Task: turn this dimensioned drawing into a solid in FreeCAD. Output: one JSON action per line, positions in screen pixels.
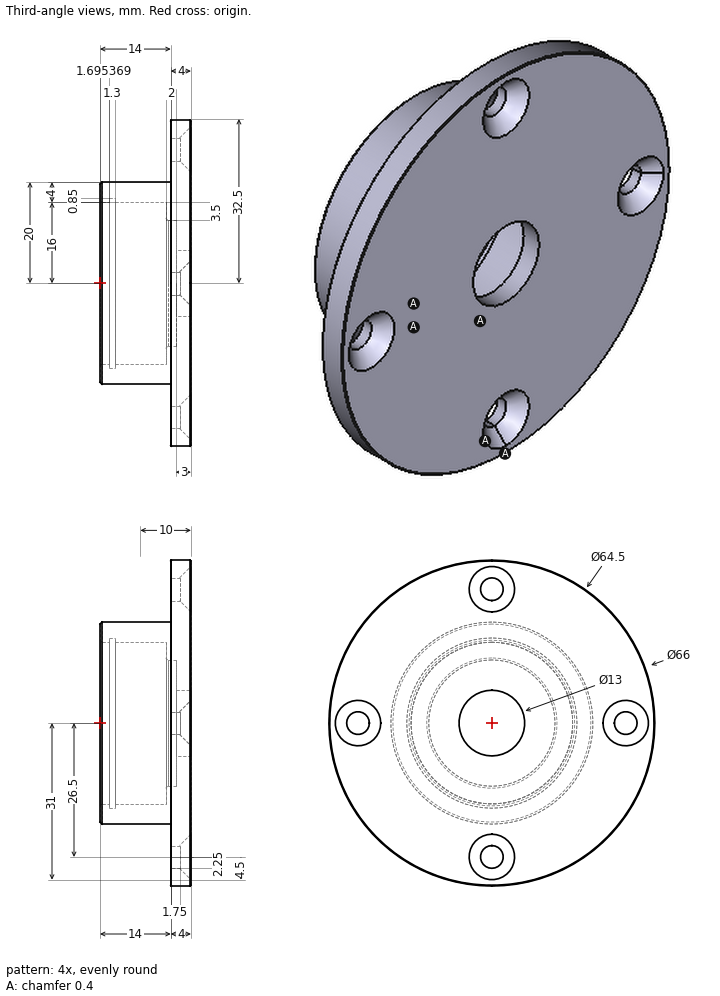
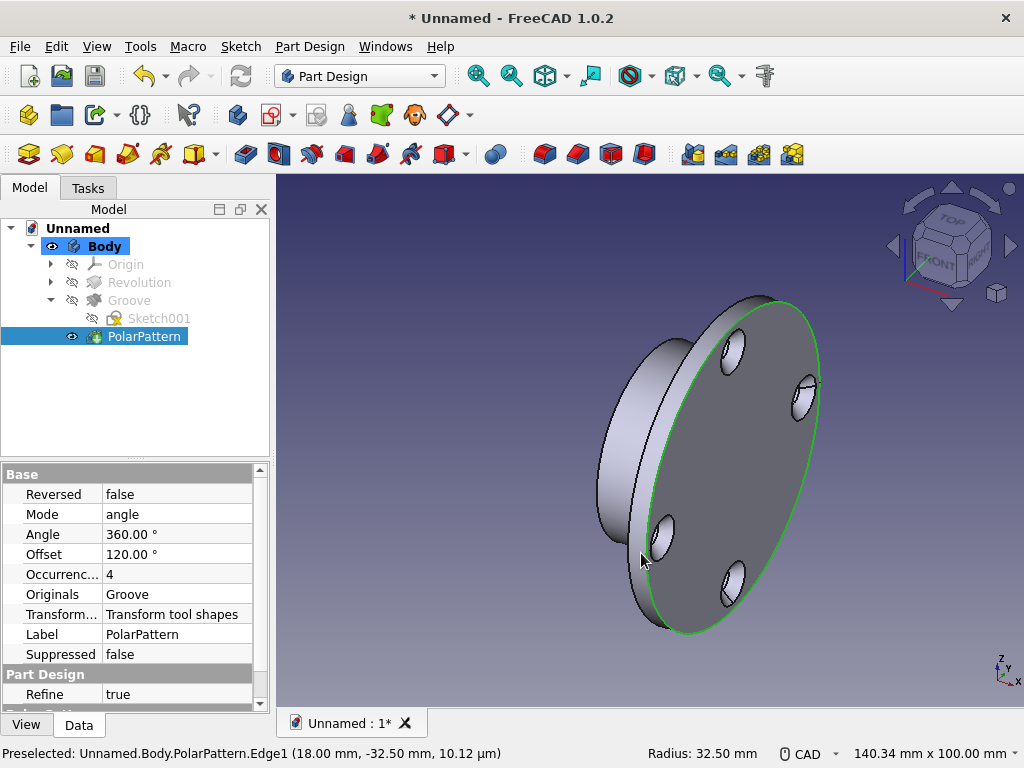
{"action": "key", "text": "0"}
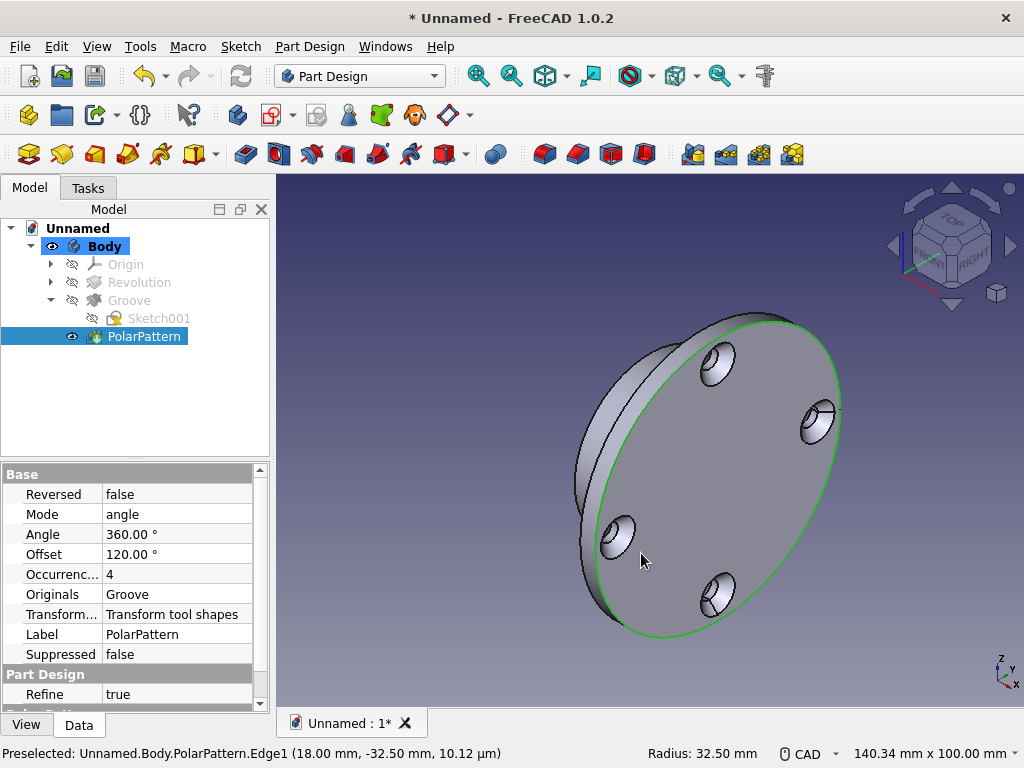
{"action": "key", "text": "2"}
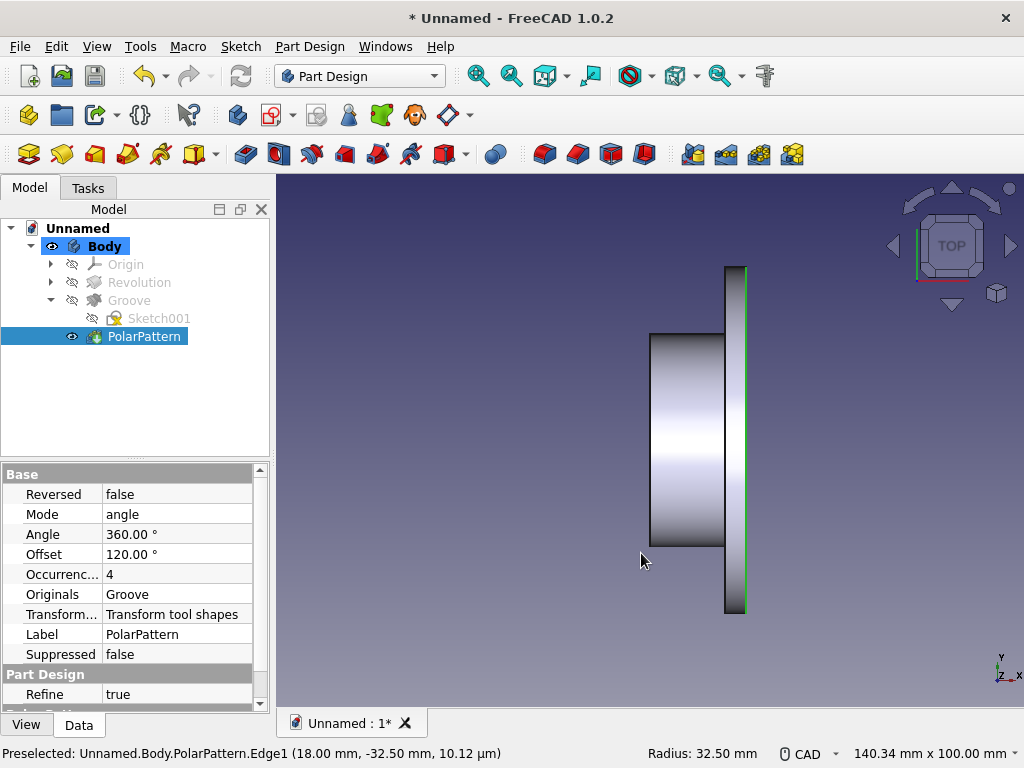
{"action": "left_click", "coordinate": [725, 580], "text": "ctrl"}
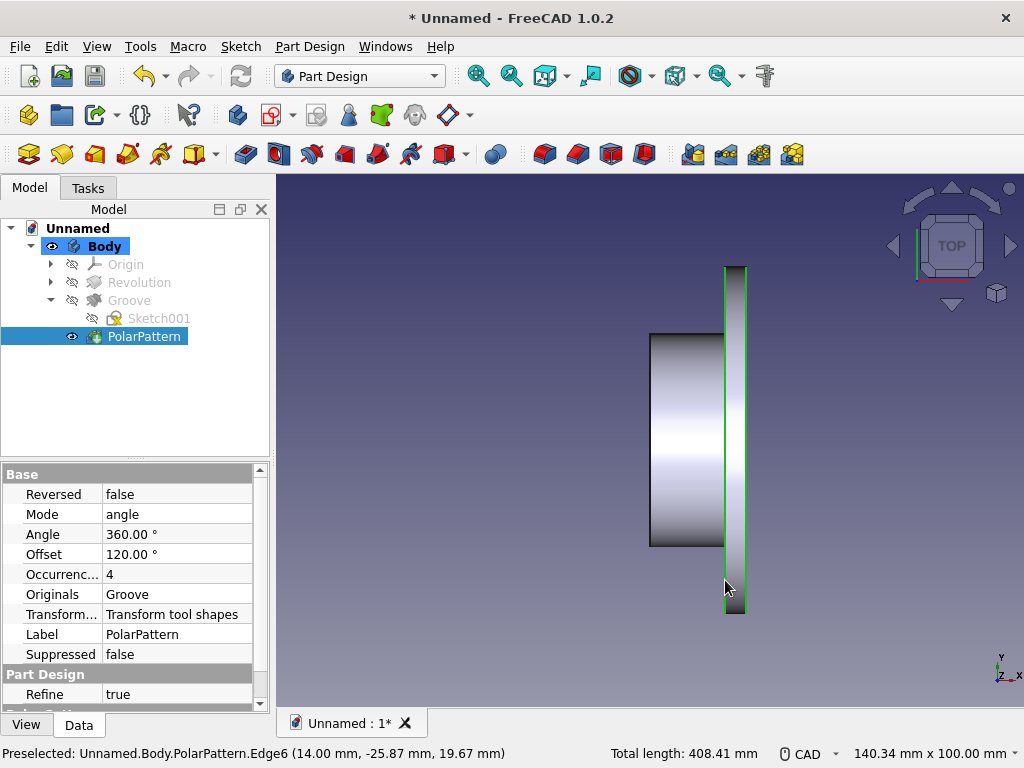
{"action": "left_click", "coordinate": [650, 526], "text": "ctrl"}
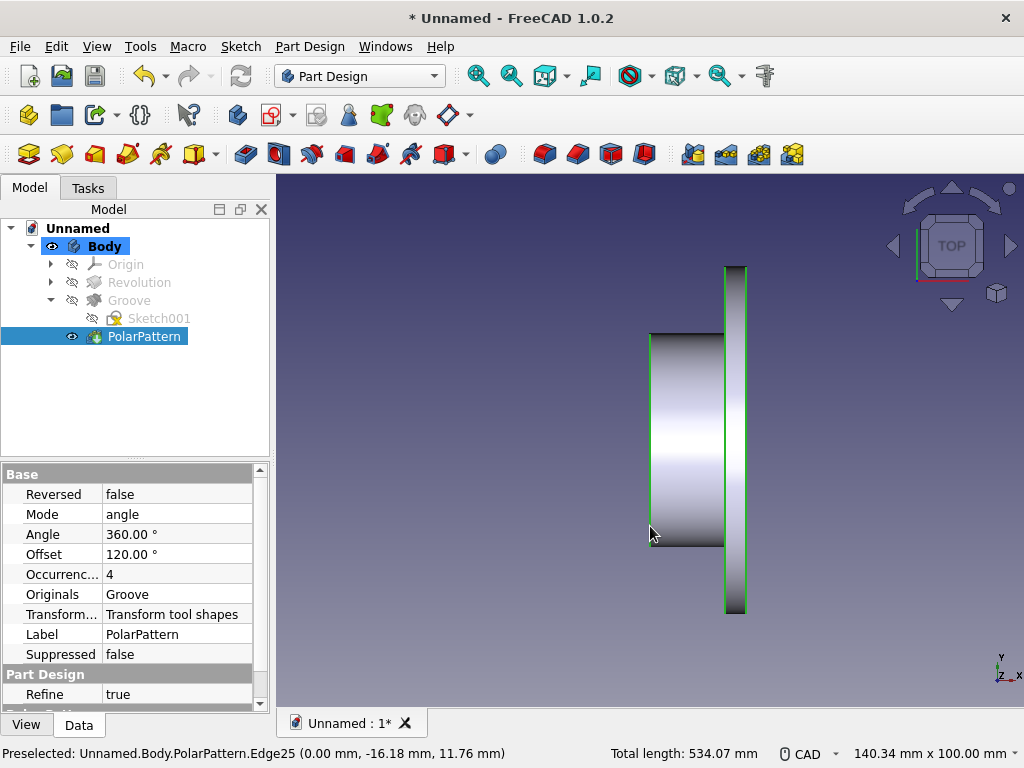
{"action": "key", "text": "1"}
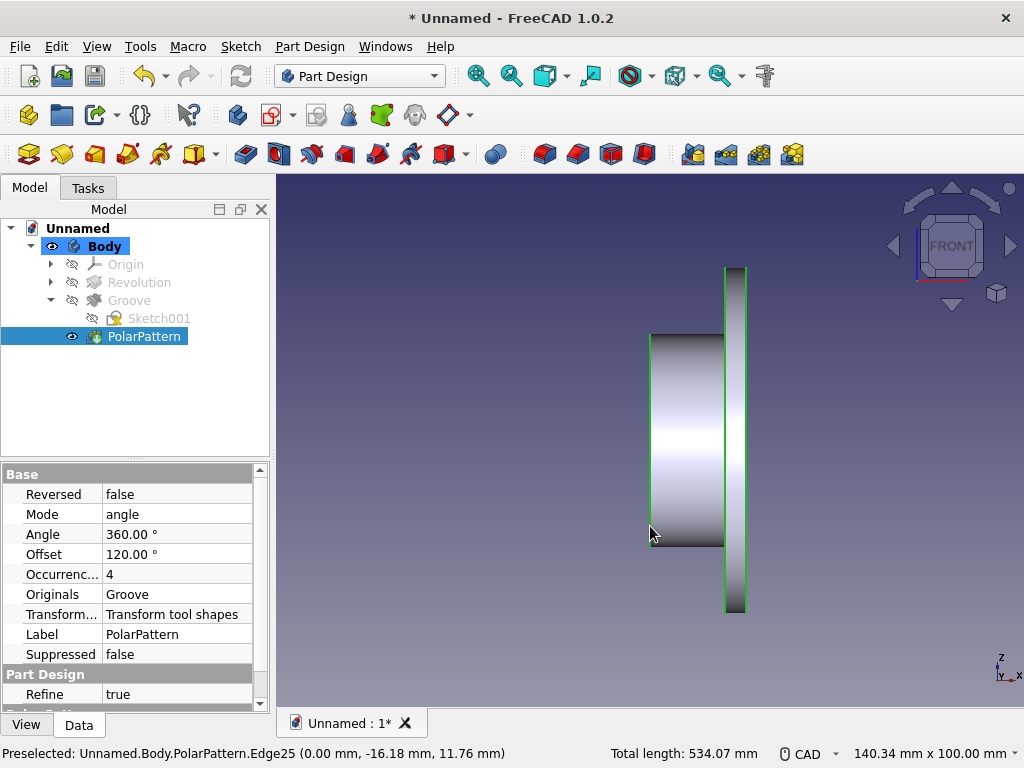
{"action": "key", "text": "3"}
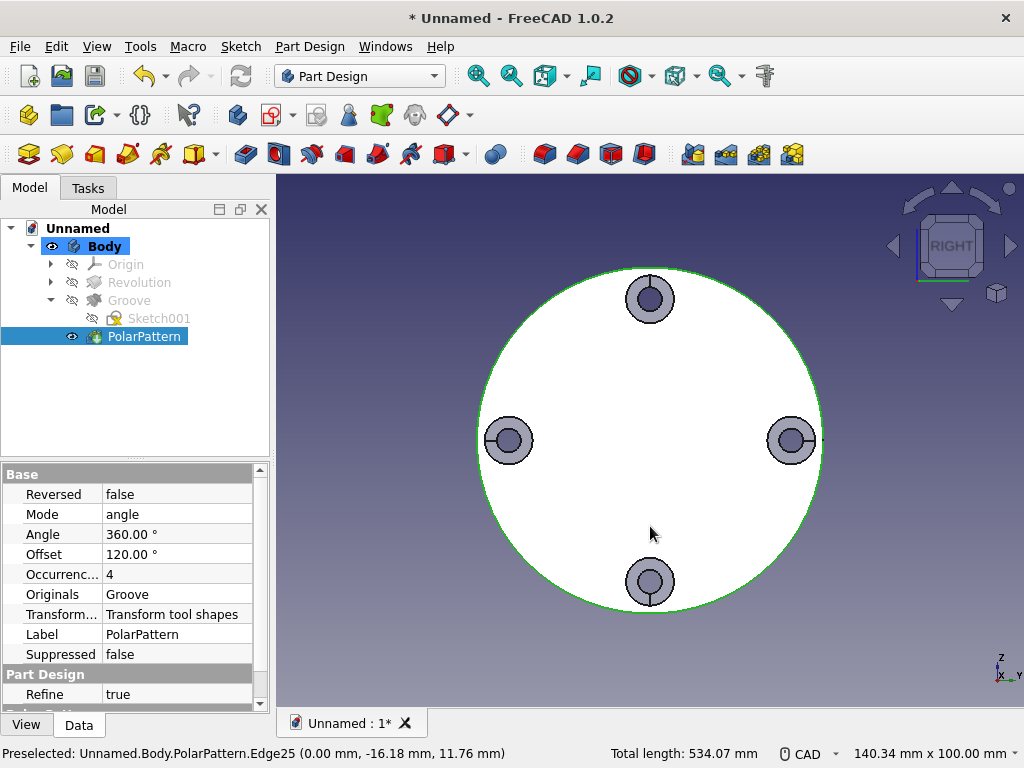
{"action": "key", "text": "5"}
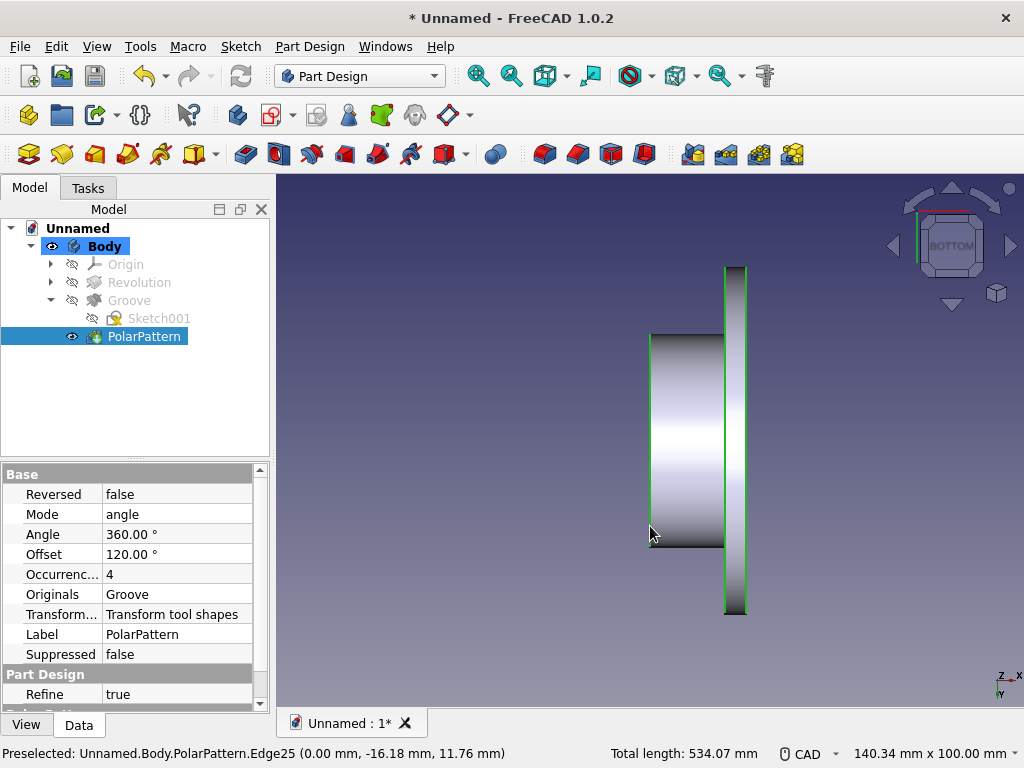
{"action": "key", "text": "4"}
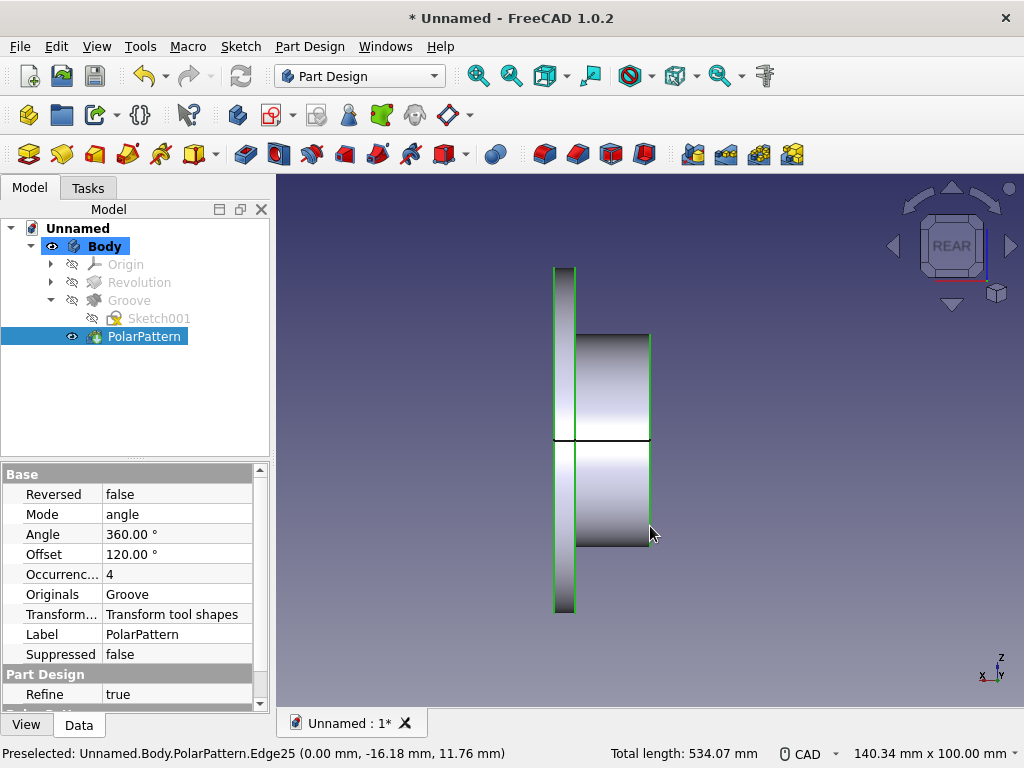
{"action": "key", "text": "6"}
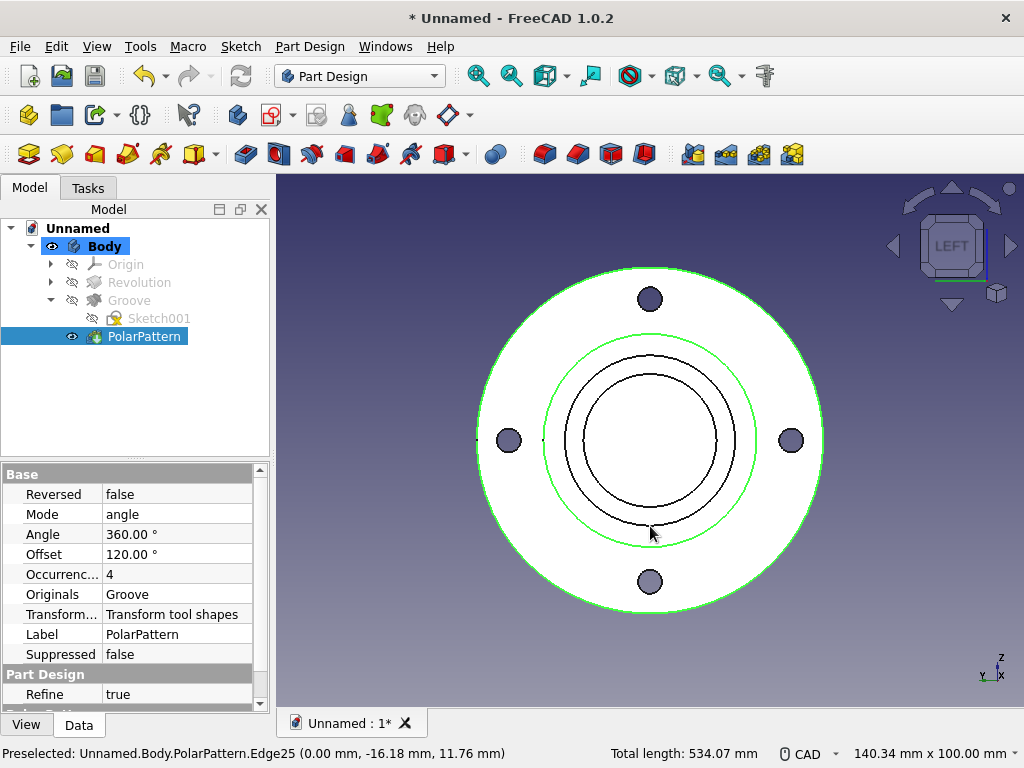
{"action": "left_click", "coordinate": [717, 439], "text": "ctrl"}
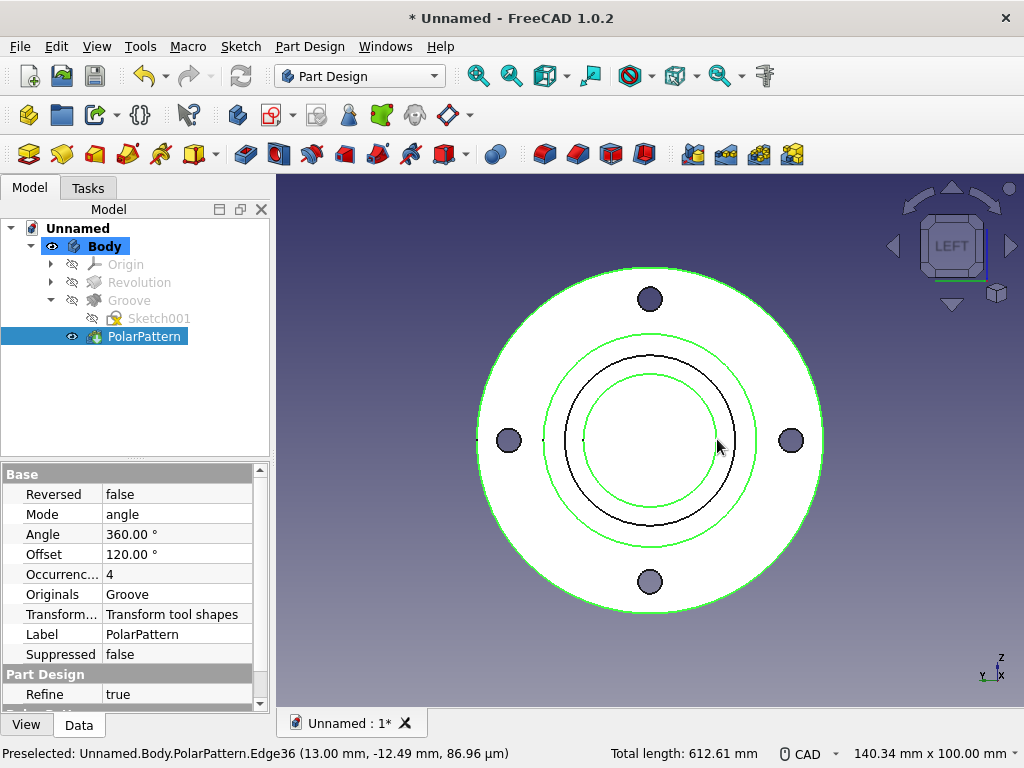
{"action": "left_click", "coordinate": [676, 358], "text": "ctrl"}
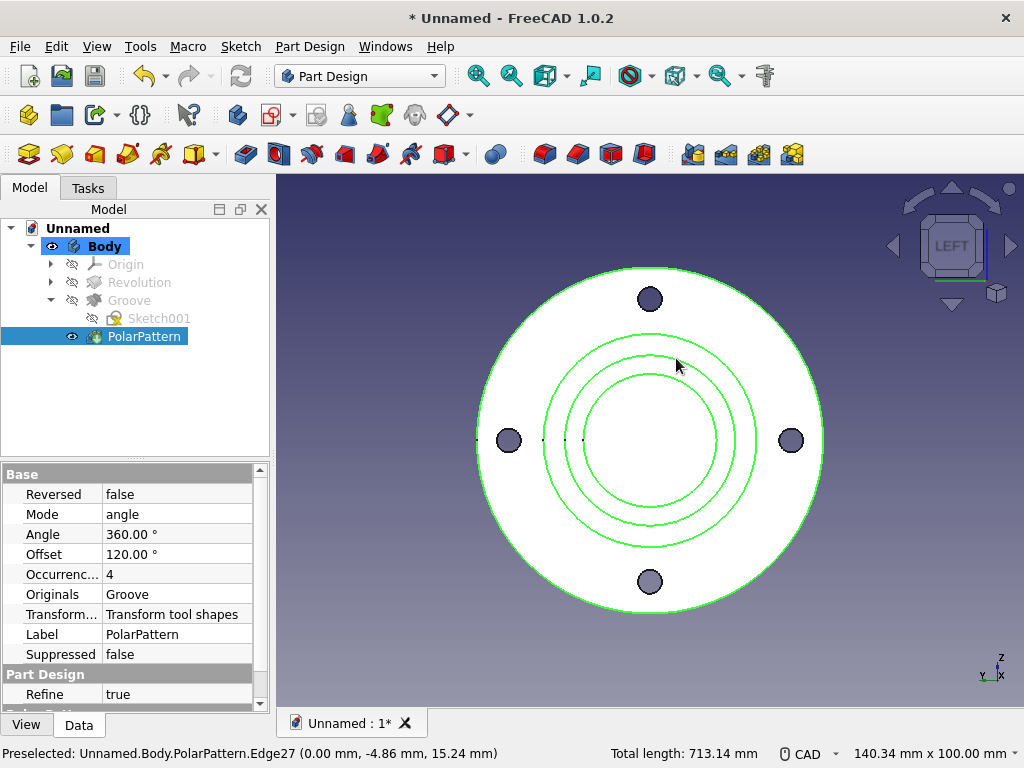
{"action": "left_click", "coordinate": [578, 154]}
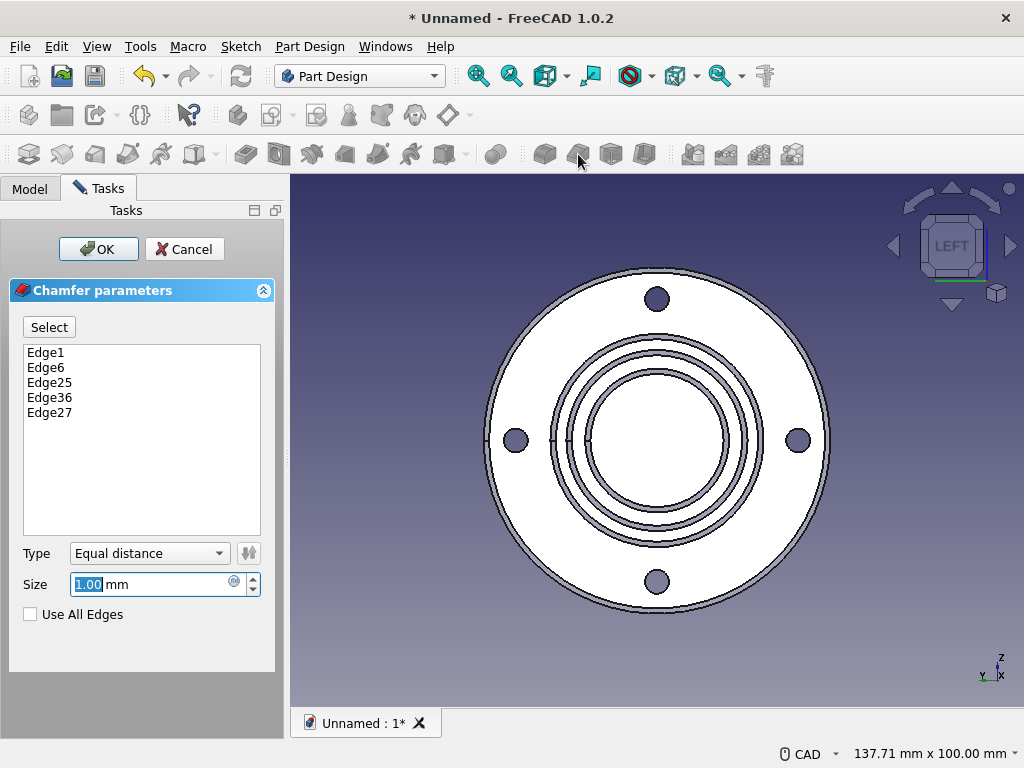
{"action": "type", "text": "0.4"}
{"action": "key", "text": "Tab"}